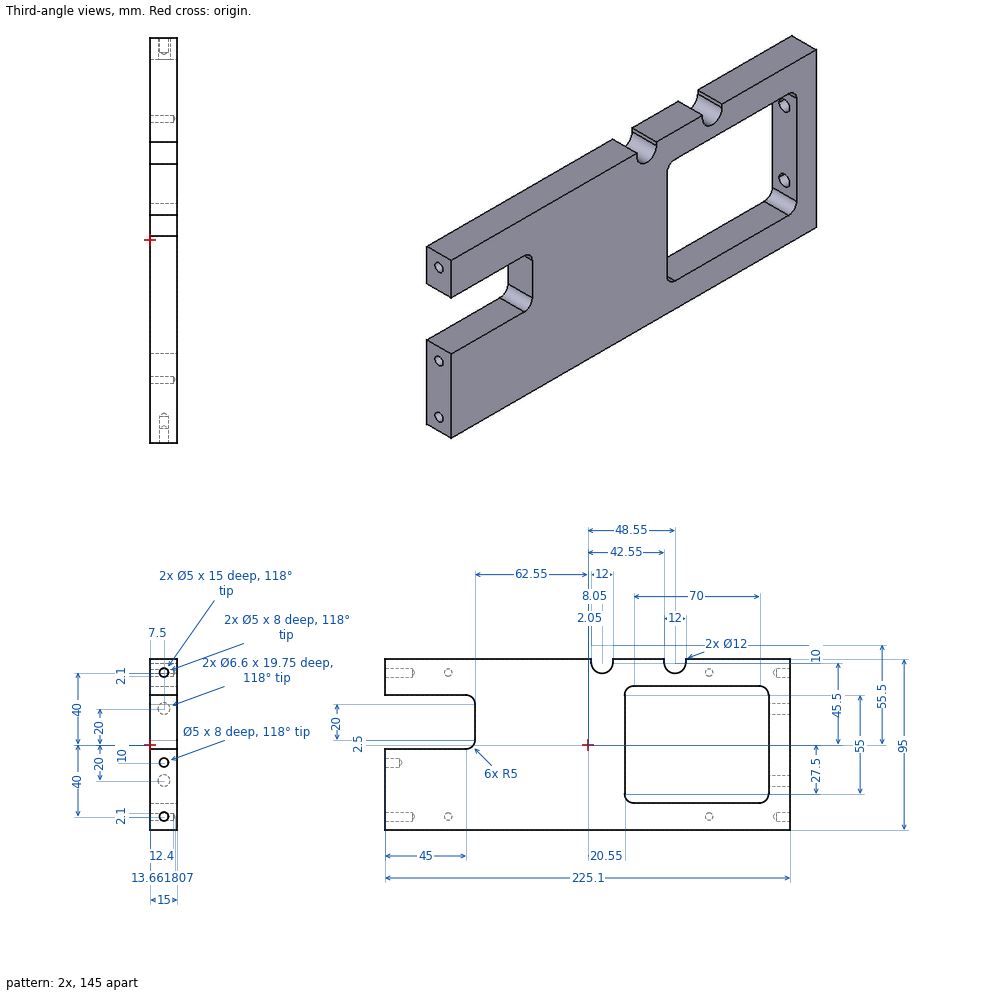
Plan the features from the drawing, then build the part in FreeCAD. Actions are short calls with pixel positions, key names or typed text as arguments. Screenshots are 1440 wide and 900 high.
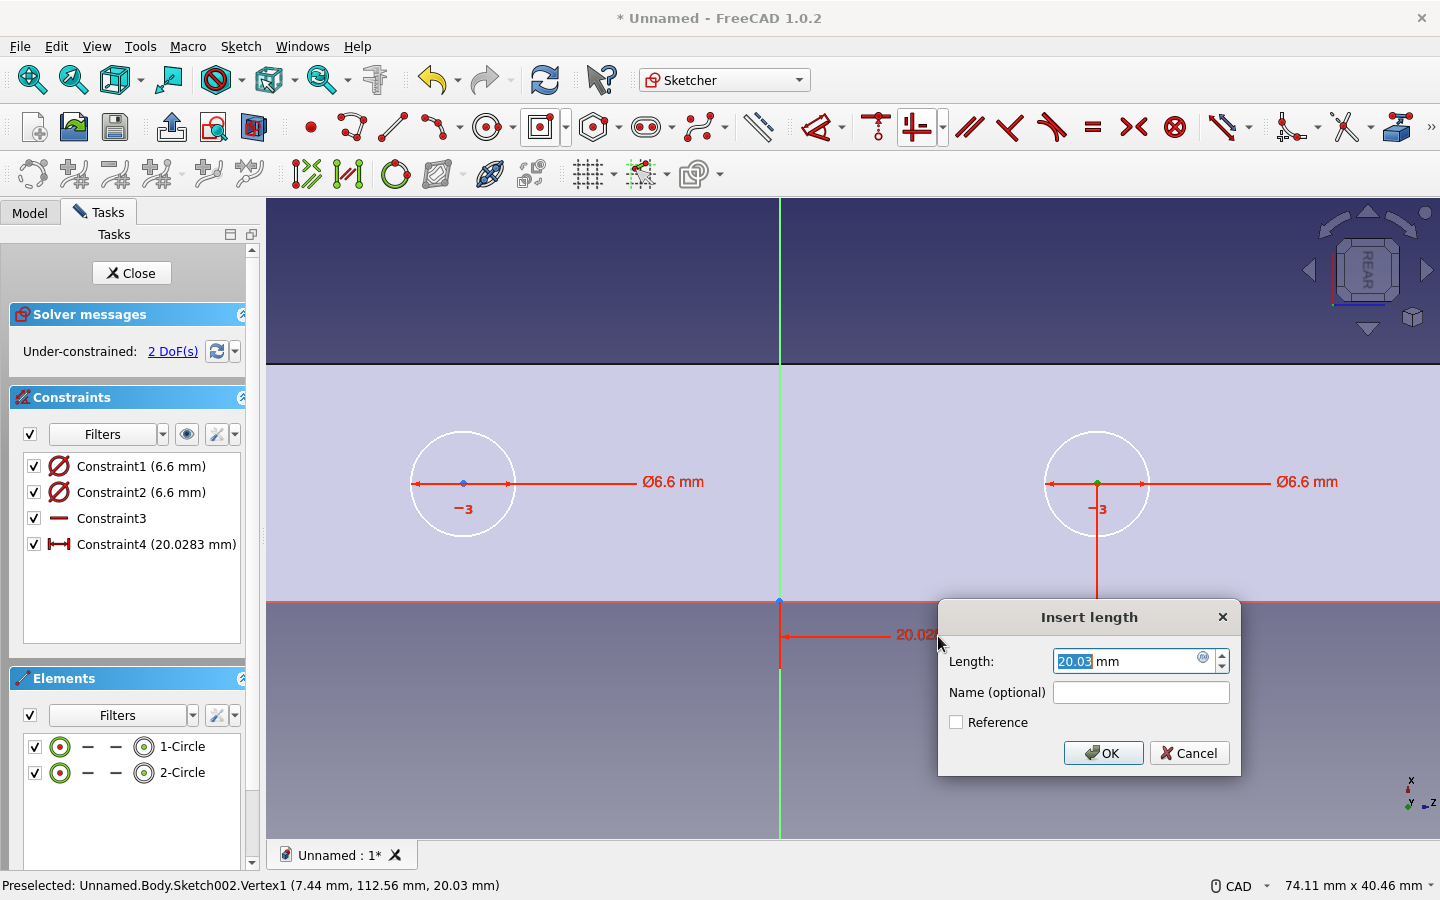
text(20)
key(Return)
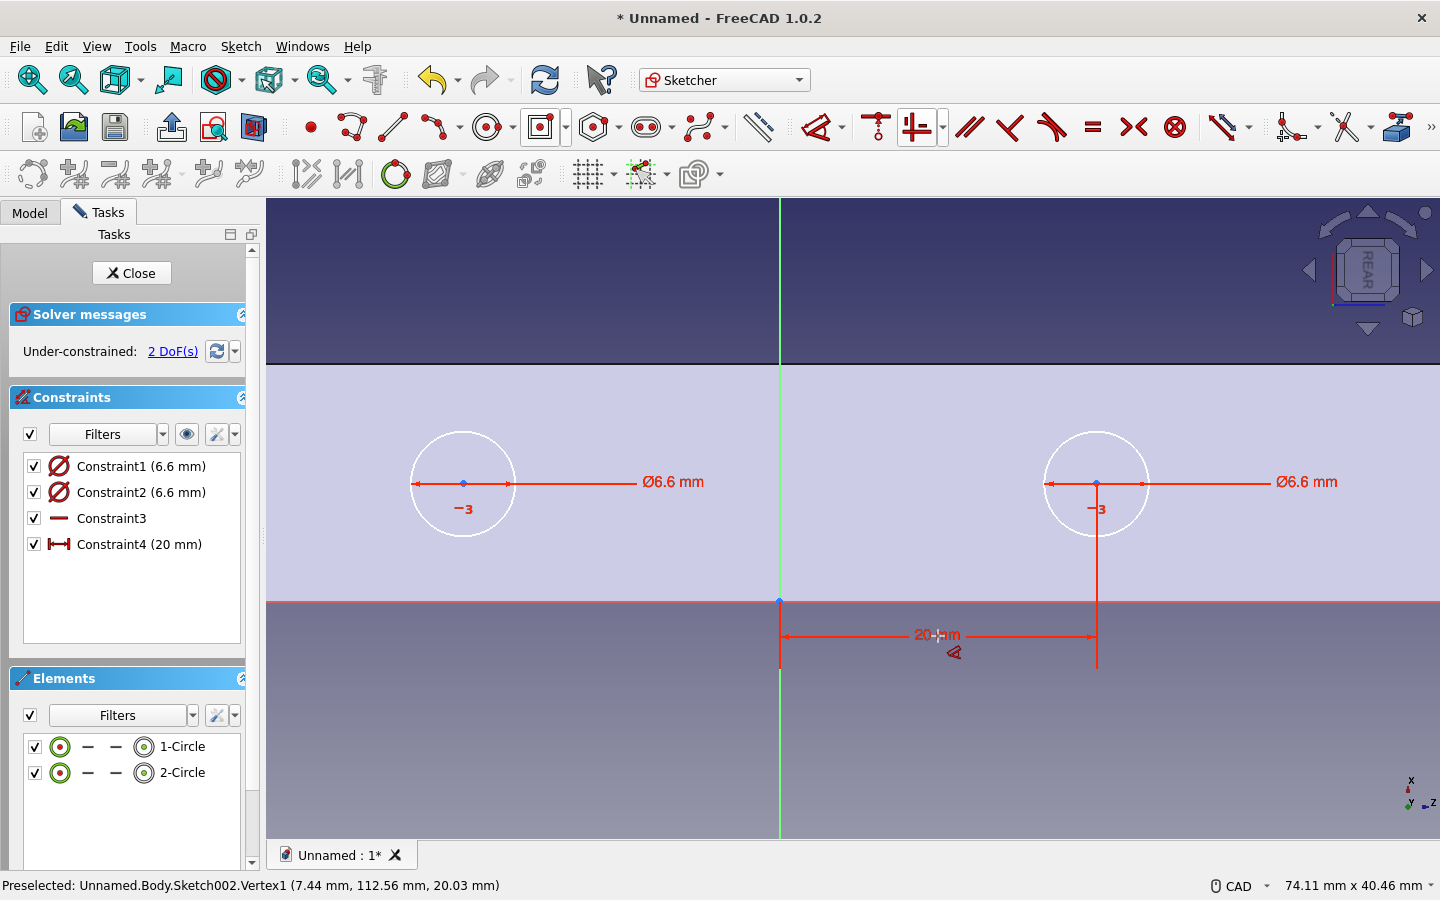
click(463, 484)
click(621, 636)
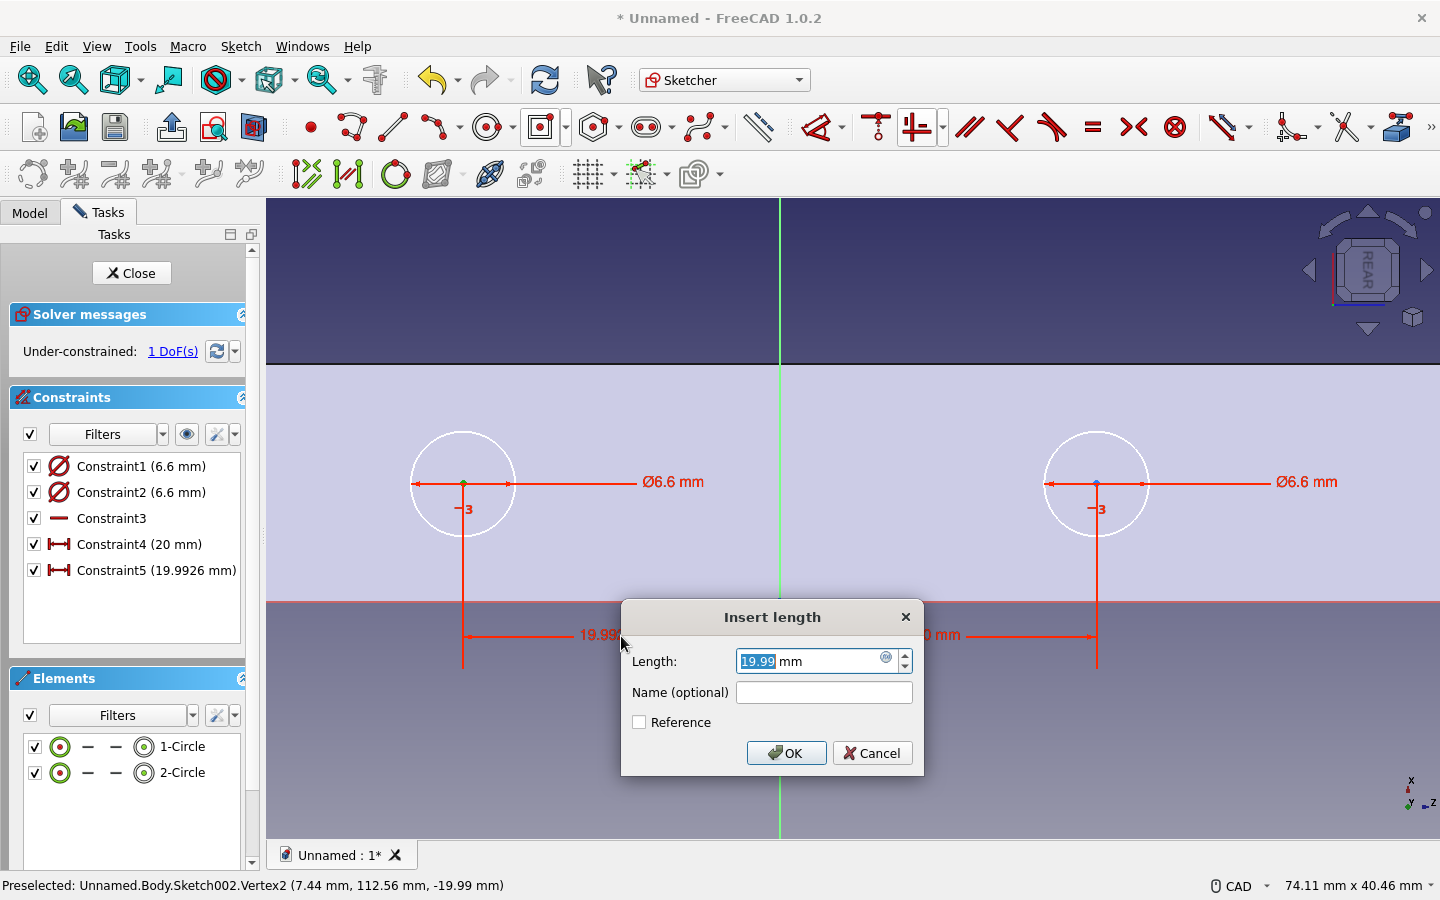
text(20)
key(Return)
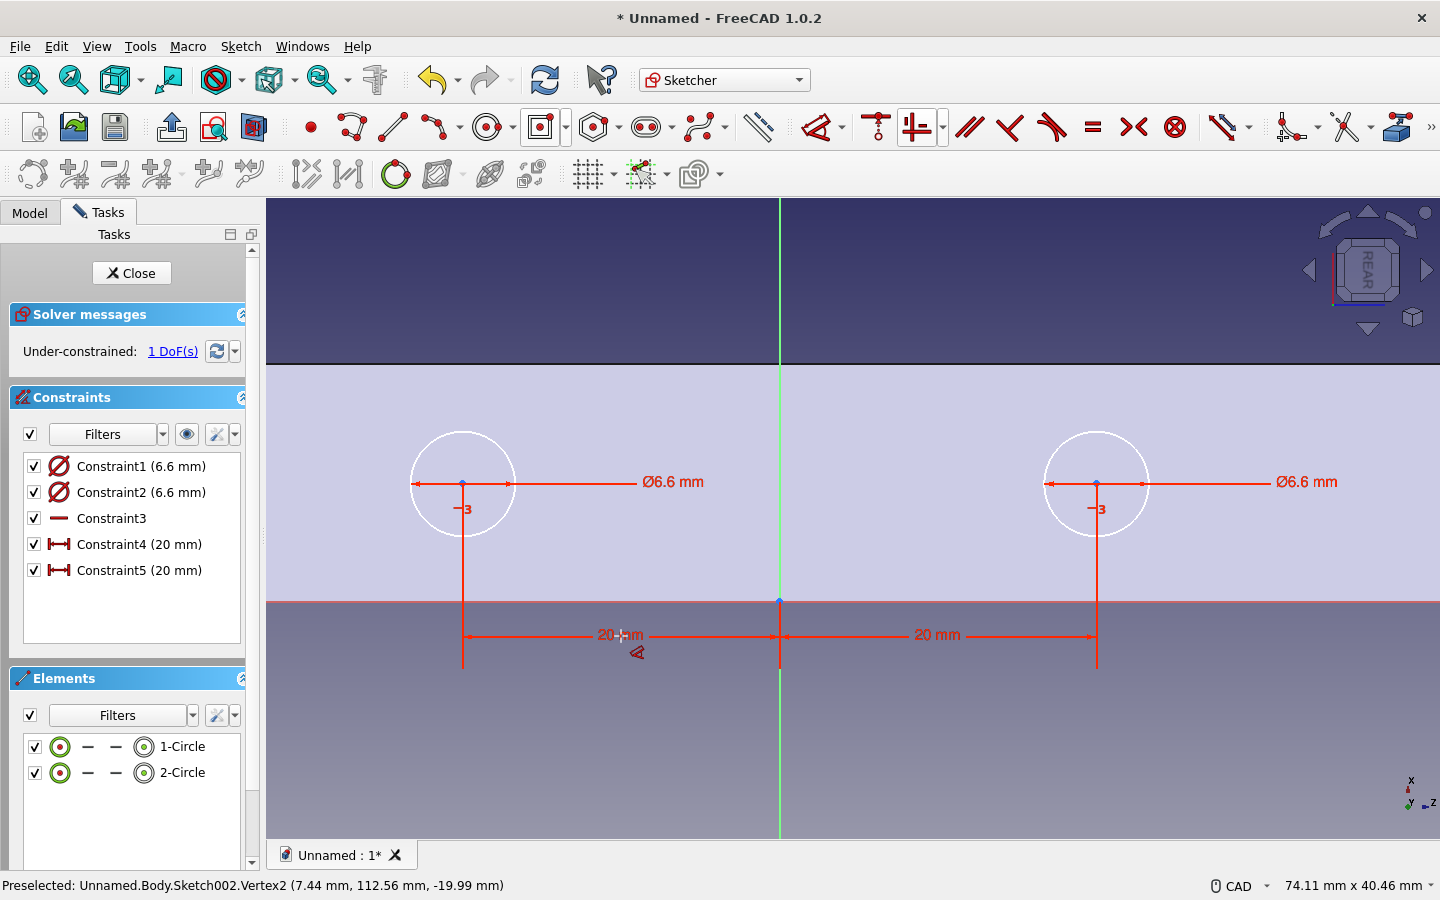
click(1097, 484)
click(1131, 543)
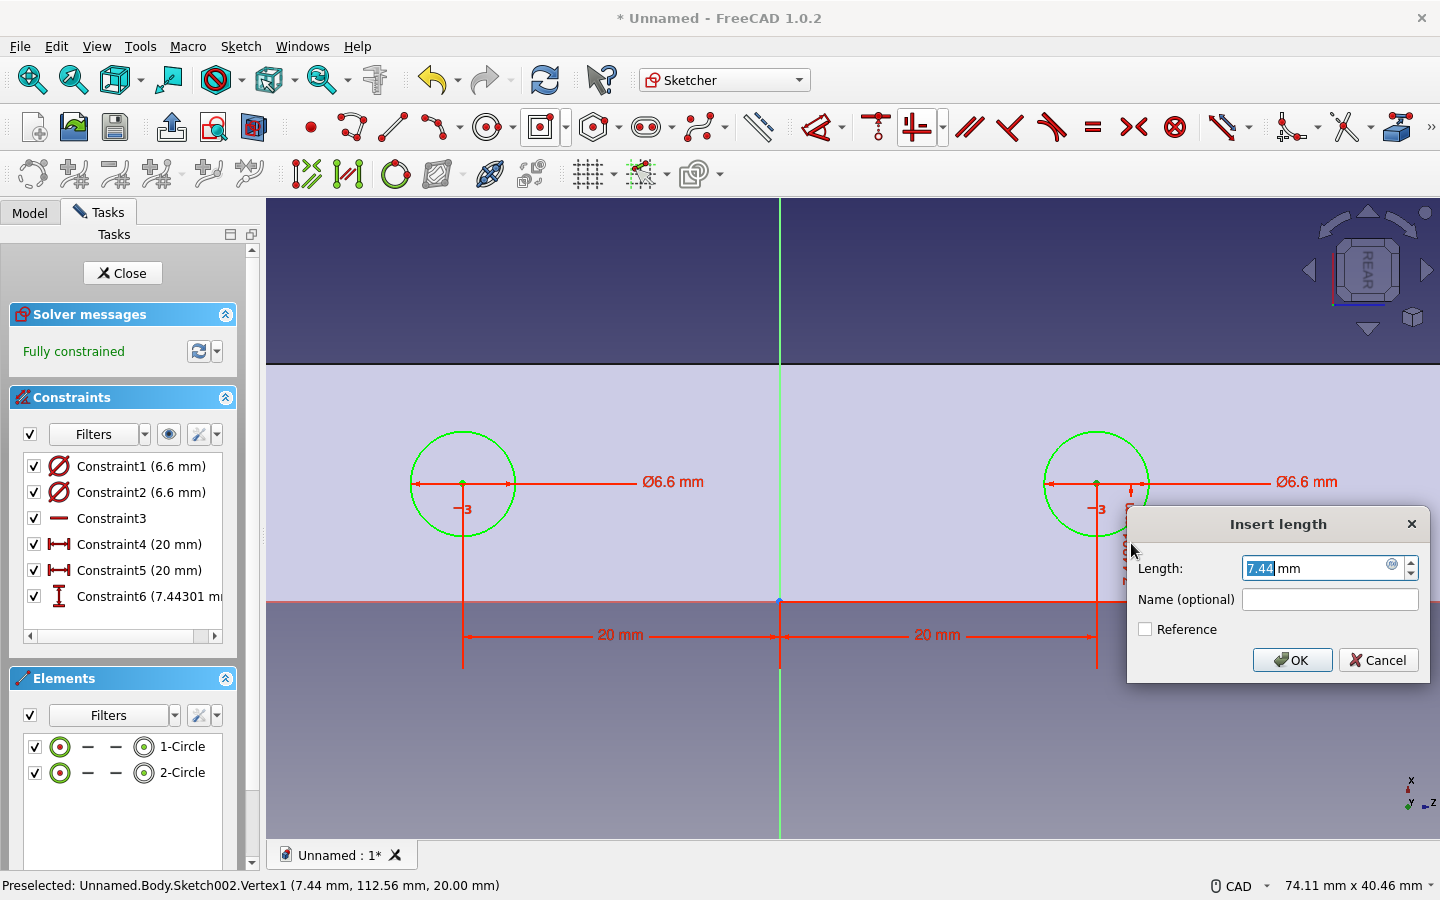
text(7.5)
key(Return)
key(Escape)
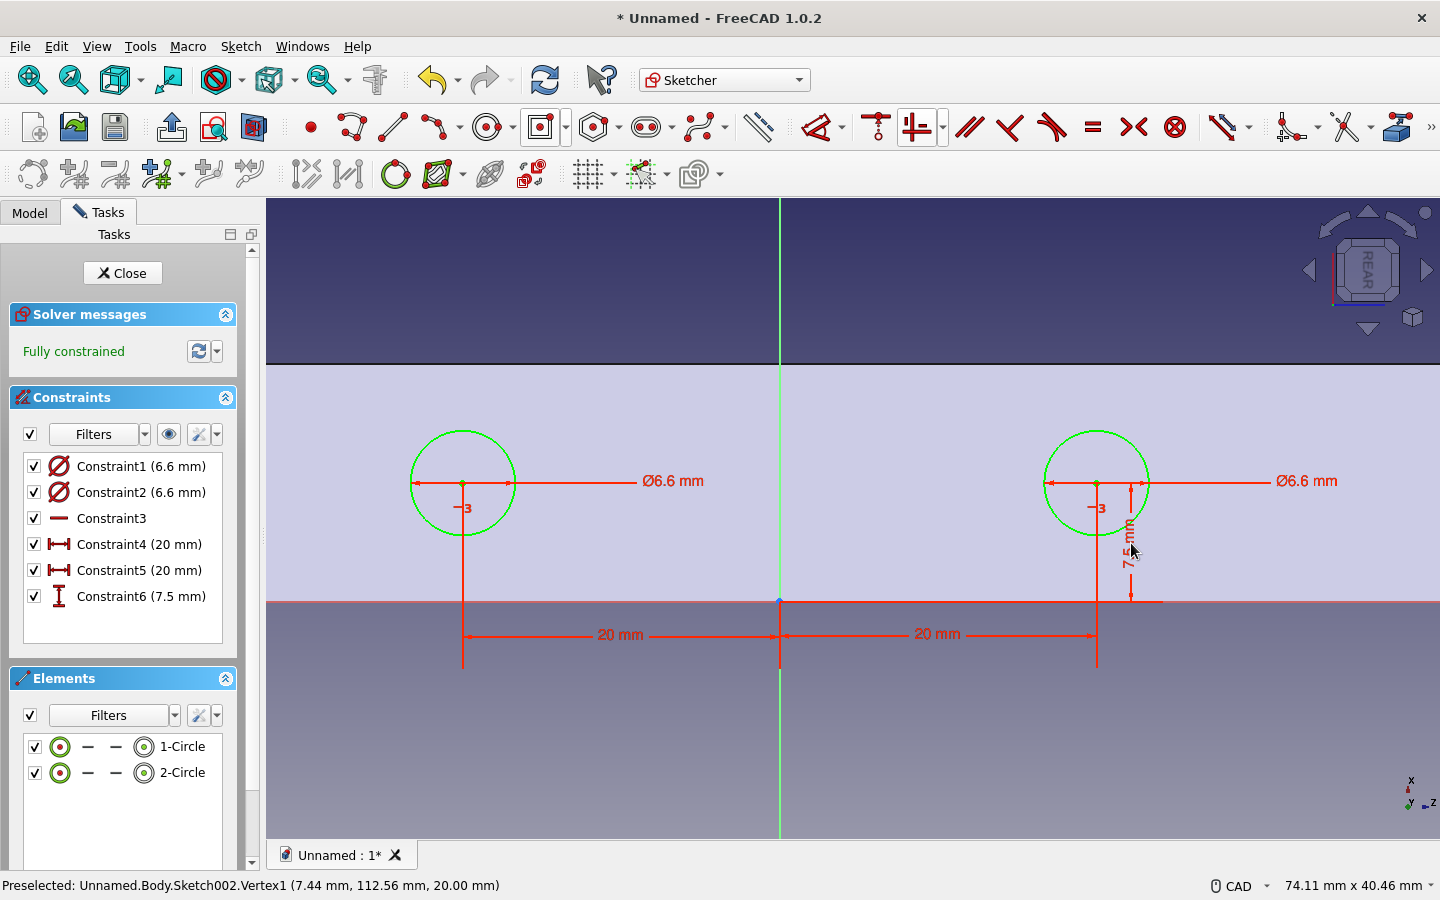
click(123, 273)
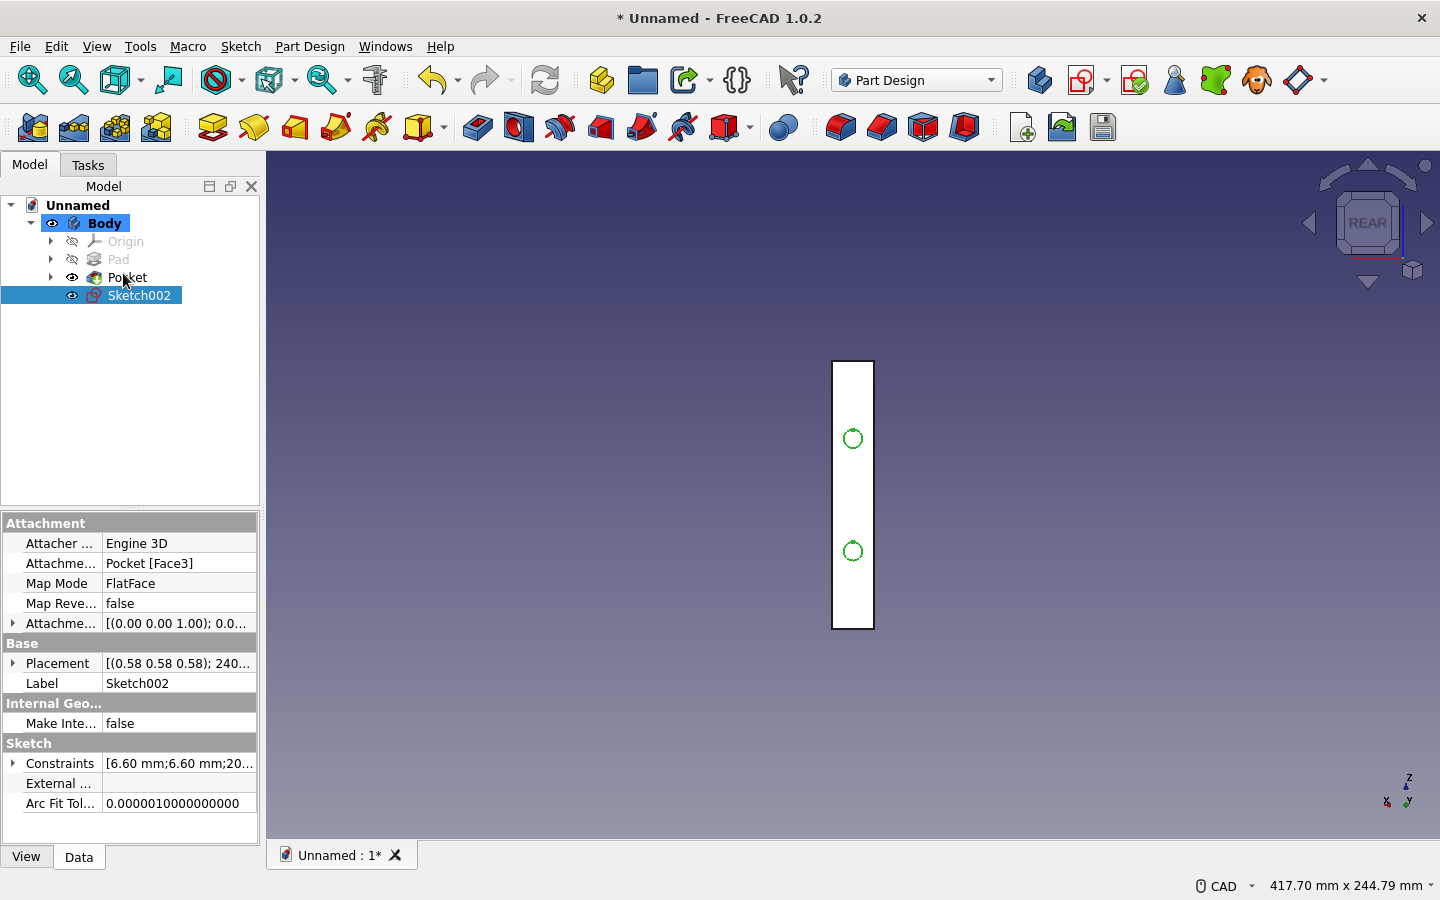
click(519, 128)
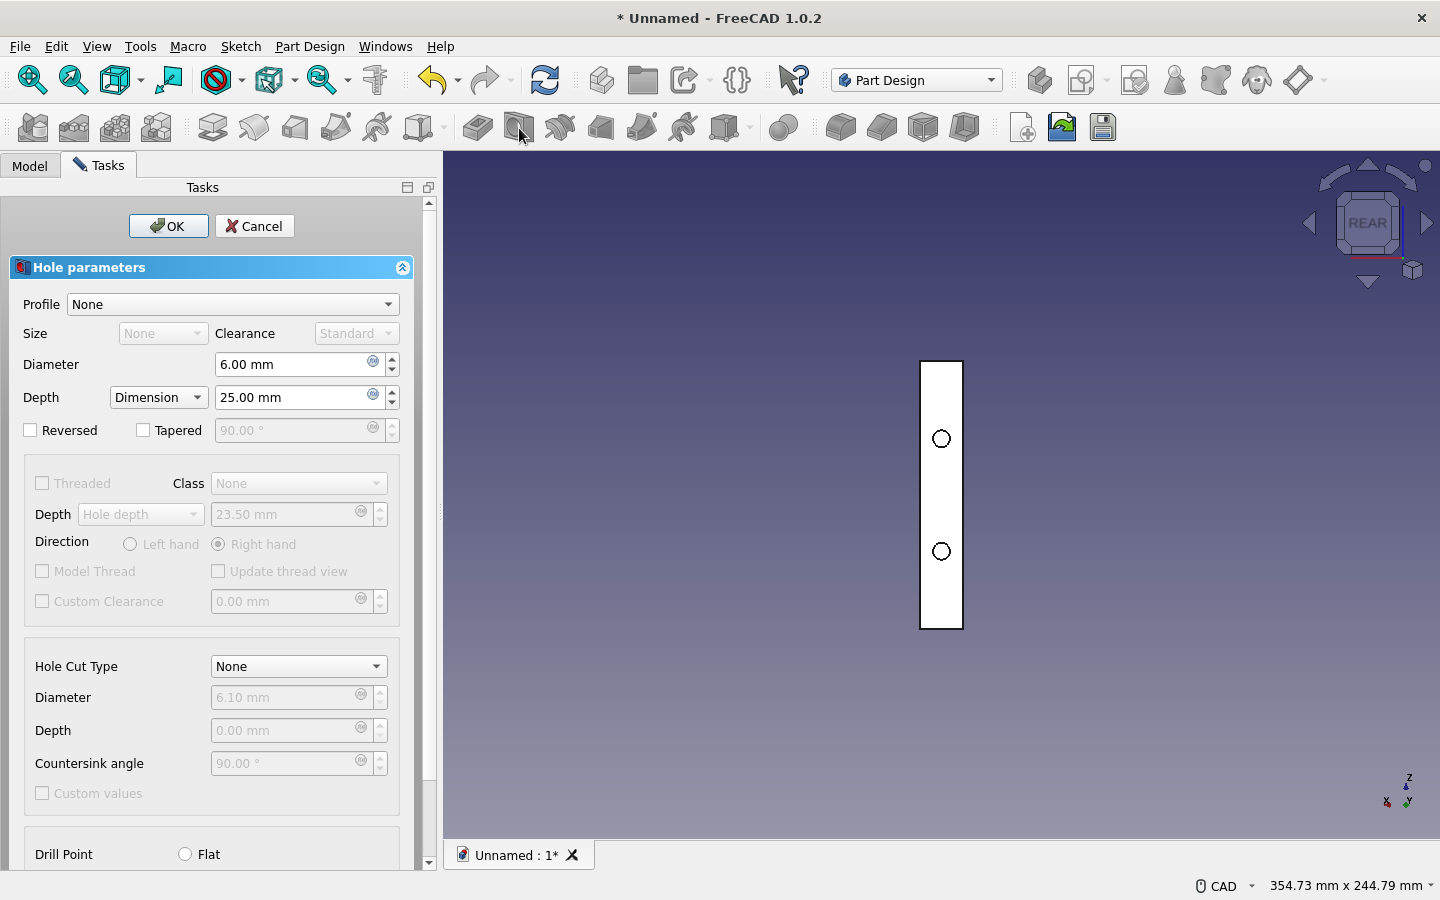
triple_click(300, 364)